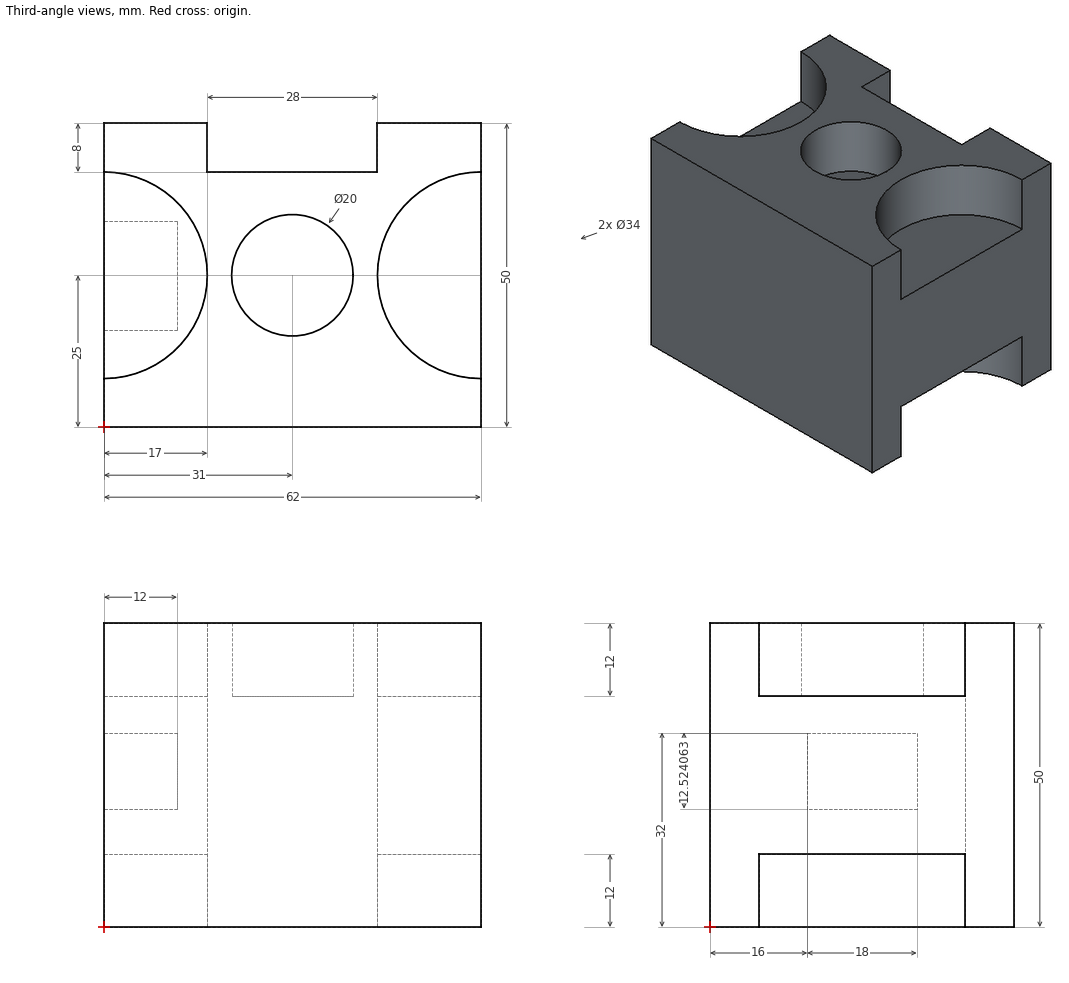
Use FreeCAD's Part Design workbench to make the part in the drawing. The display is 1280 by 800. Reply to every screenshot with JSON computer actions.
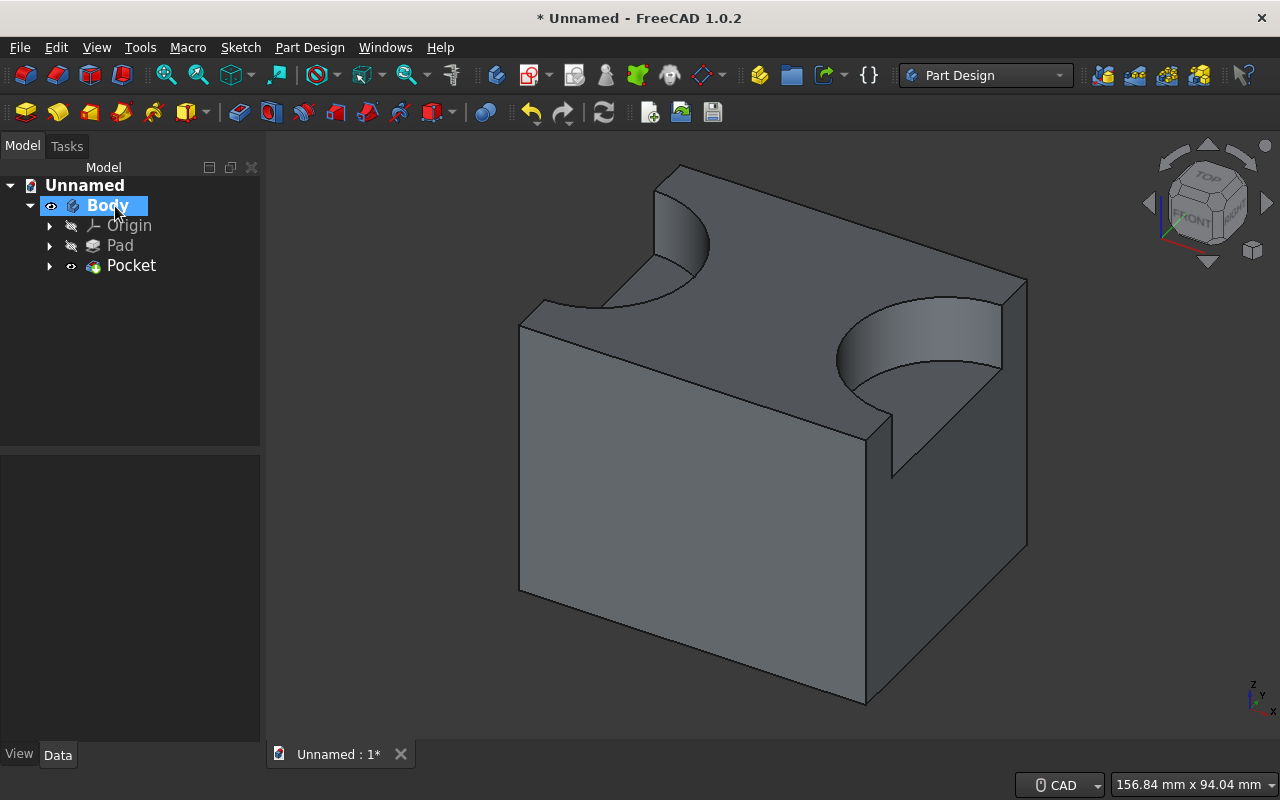
{"action": "left_click", "coordinate": [796, 279]}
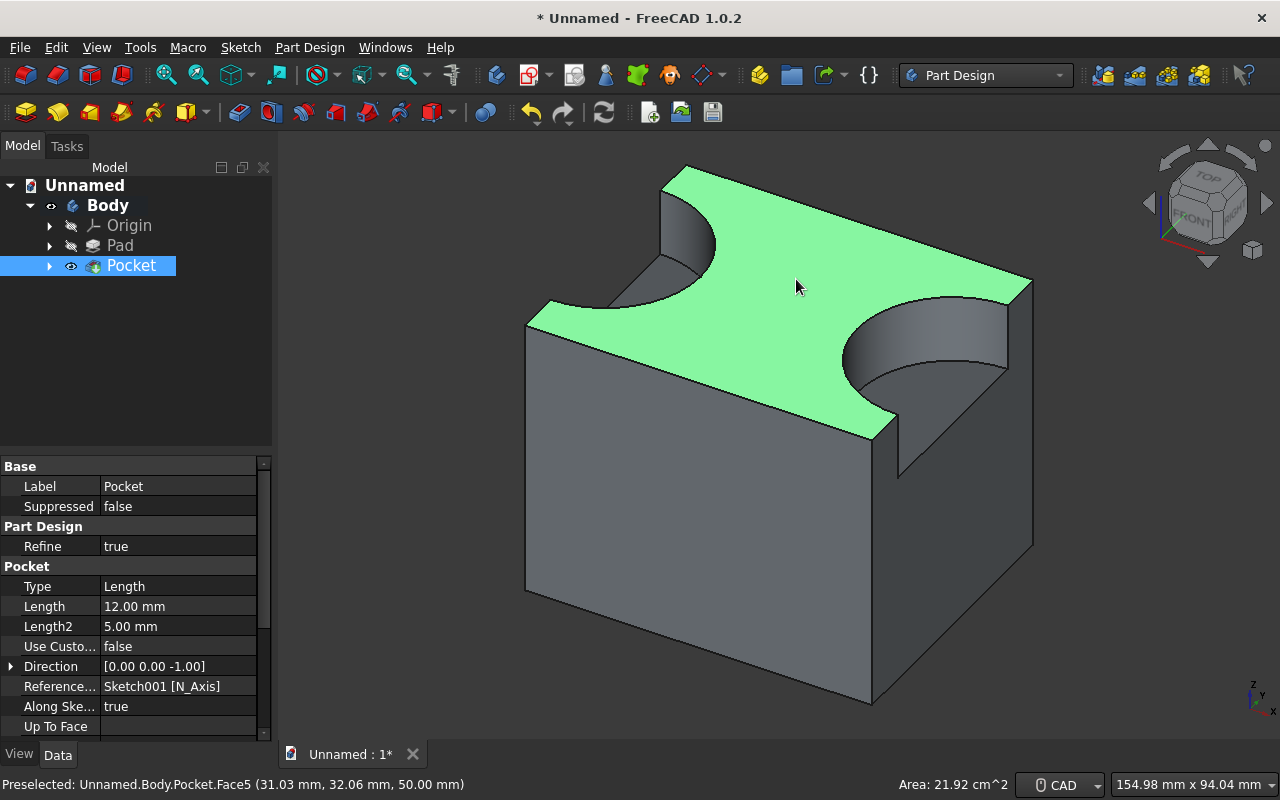
{"action": "left_click", "coordinate": [530, 76]}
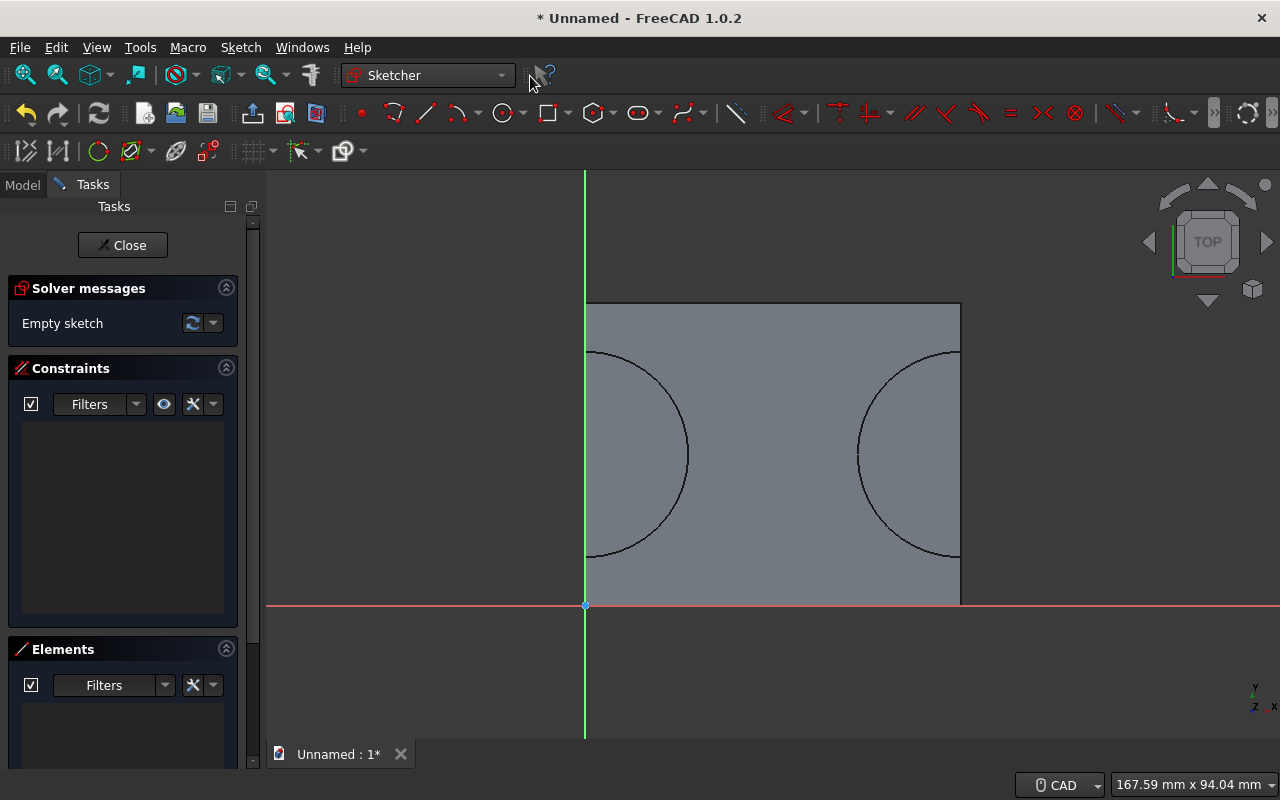
{"action": "left_click", "coordinate": [548, 114]}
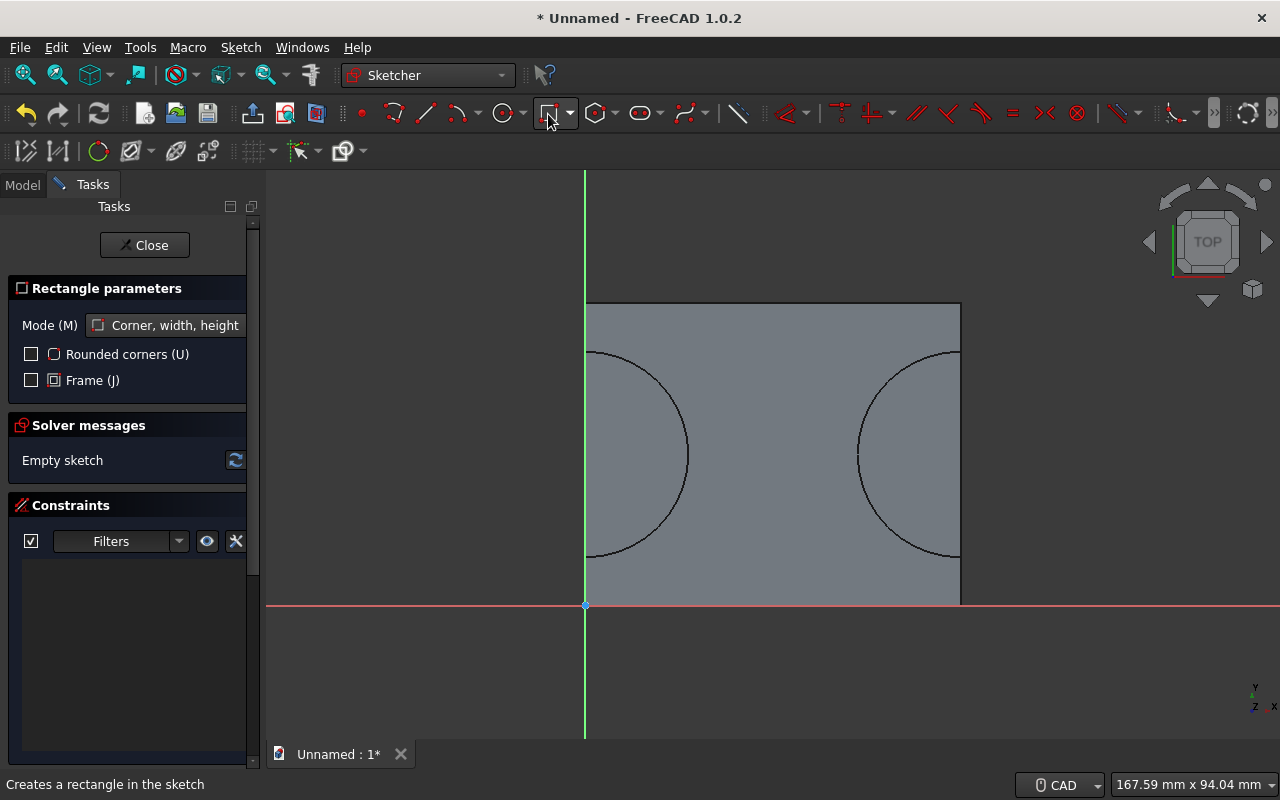
{"action": "left_click", "coordinate": [688, 303]}
{"action": "left_click", "coordinate": [858, 352]}
{"action": "key", "text": "Escape"}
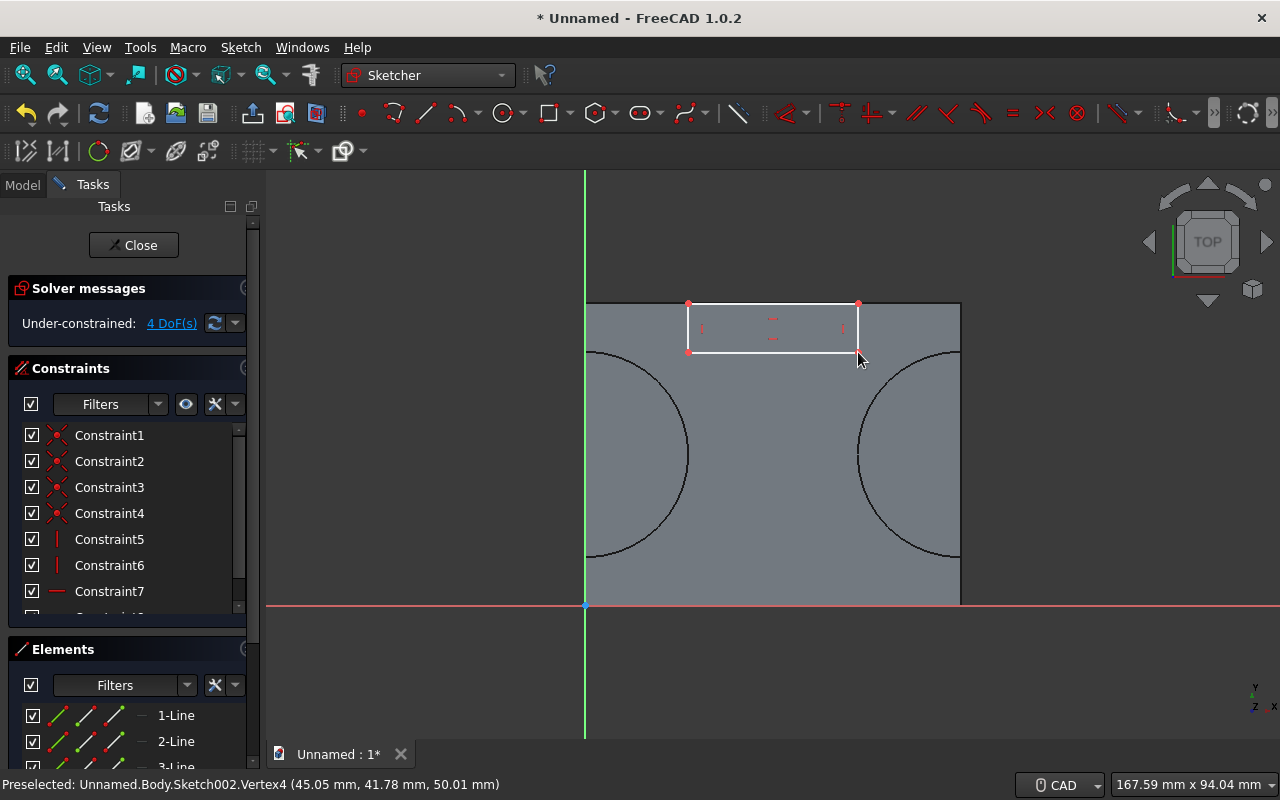
{"action": "left_click", "coordinate": [786, 114]}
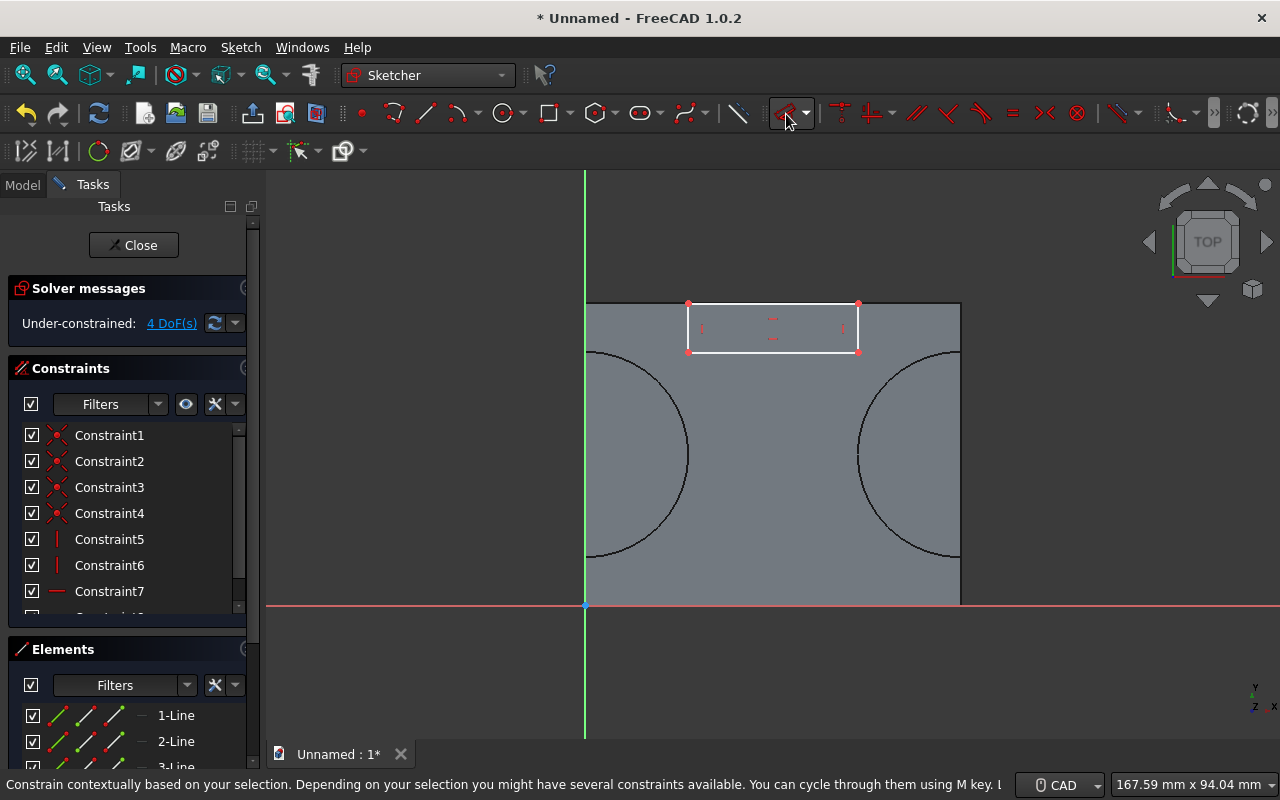
{"action": "left_click", "coordinate": [688, 319]}
{"action": "left_click", "coordinate": [654, 329]}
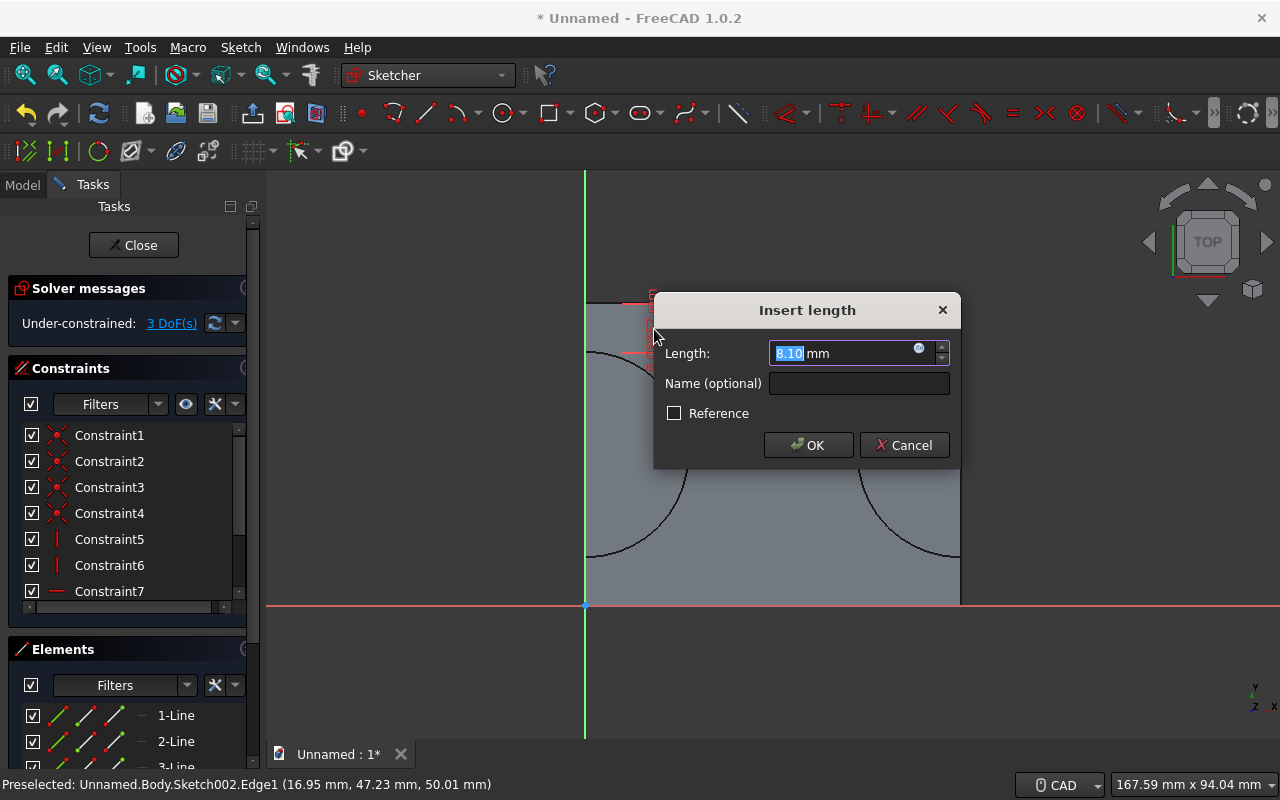
{"action": "type", "text": "8"}
{"action": "key", "text": "Return"}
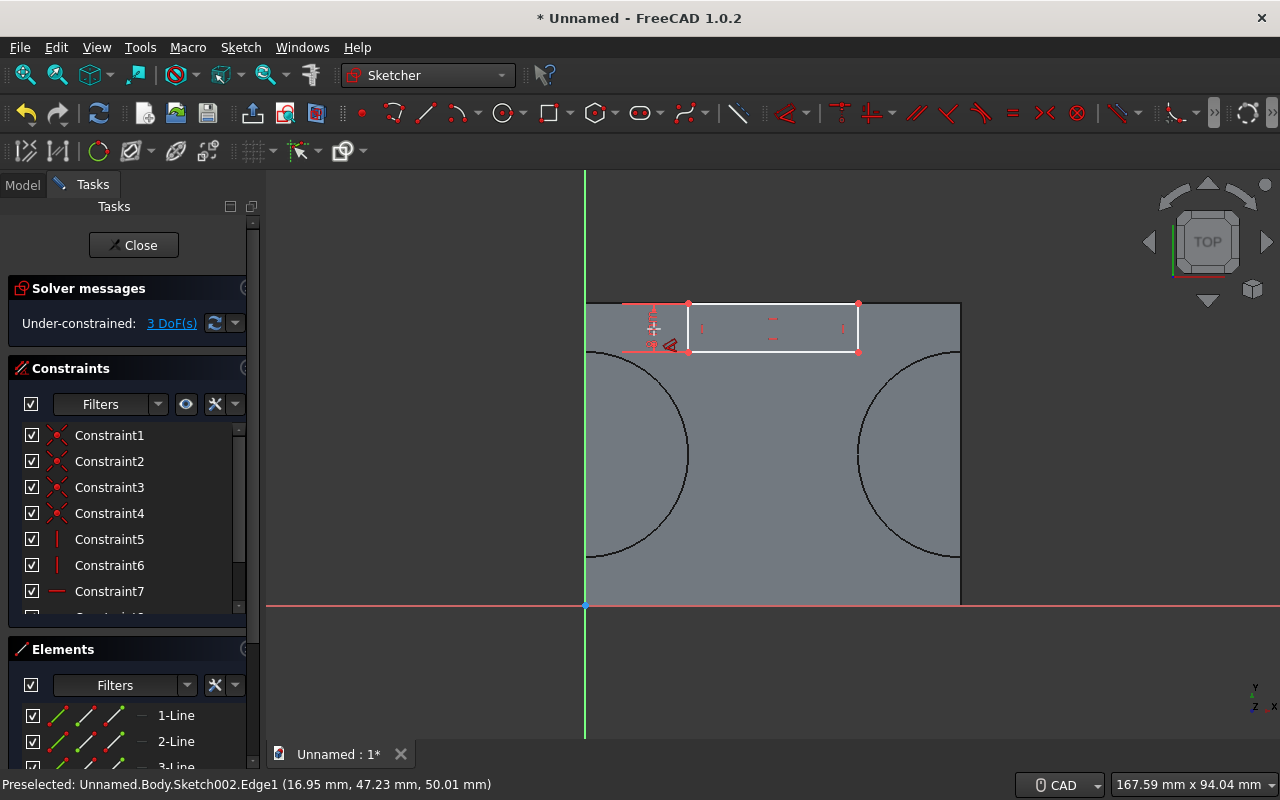
{"action": "left_click", "coordinate": [739, 352]}
{"action": "left_click", "coordinate": [773, 318]}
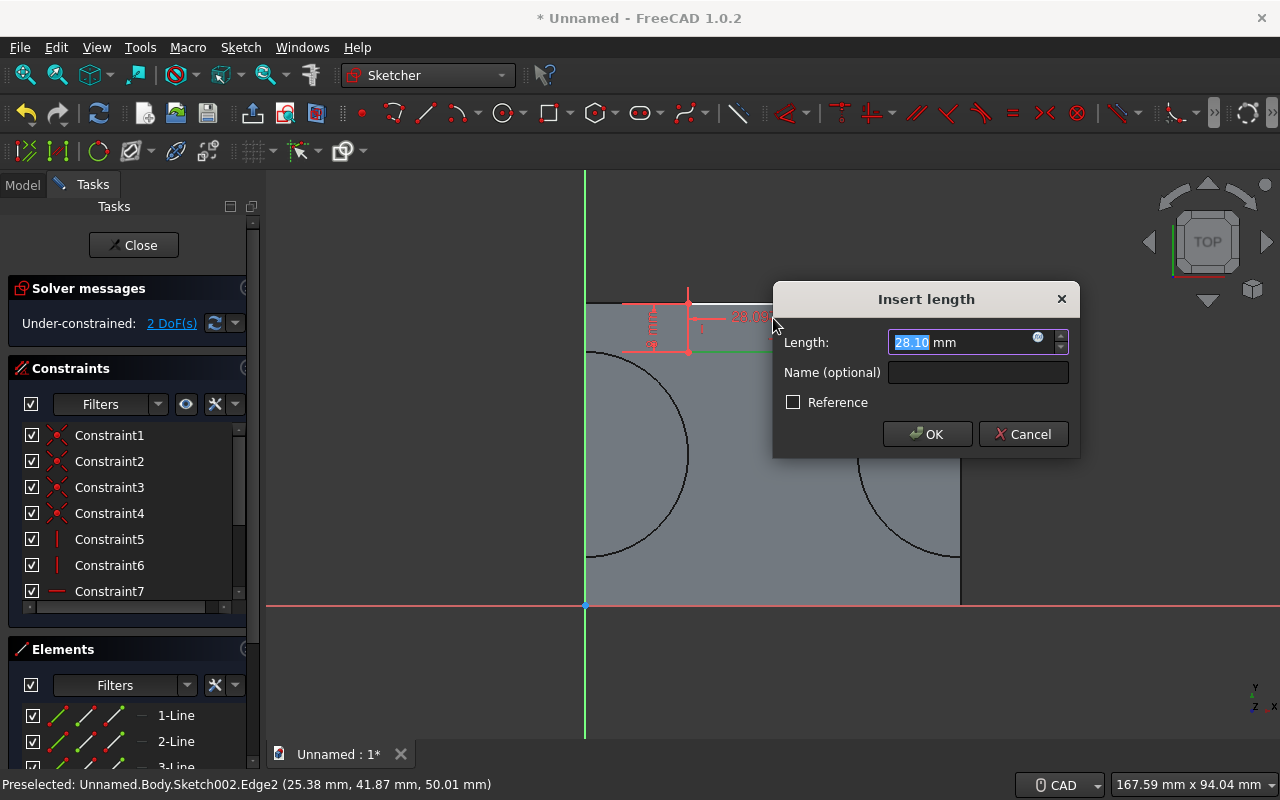
{"action": "type", "text": "28"}
{"action": "key", "text": "Return"}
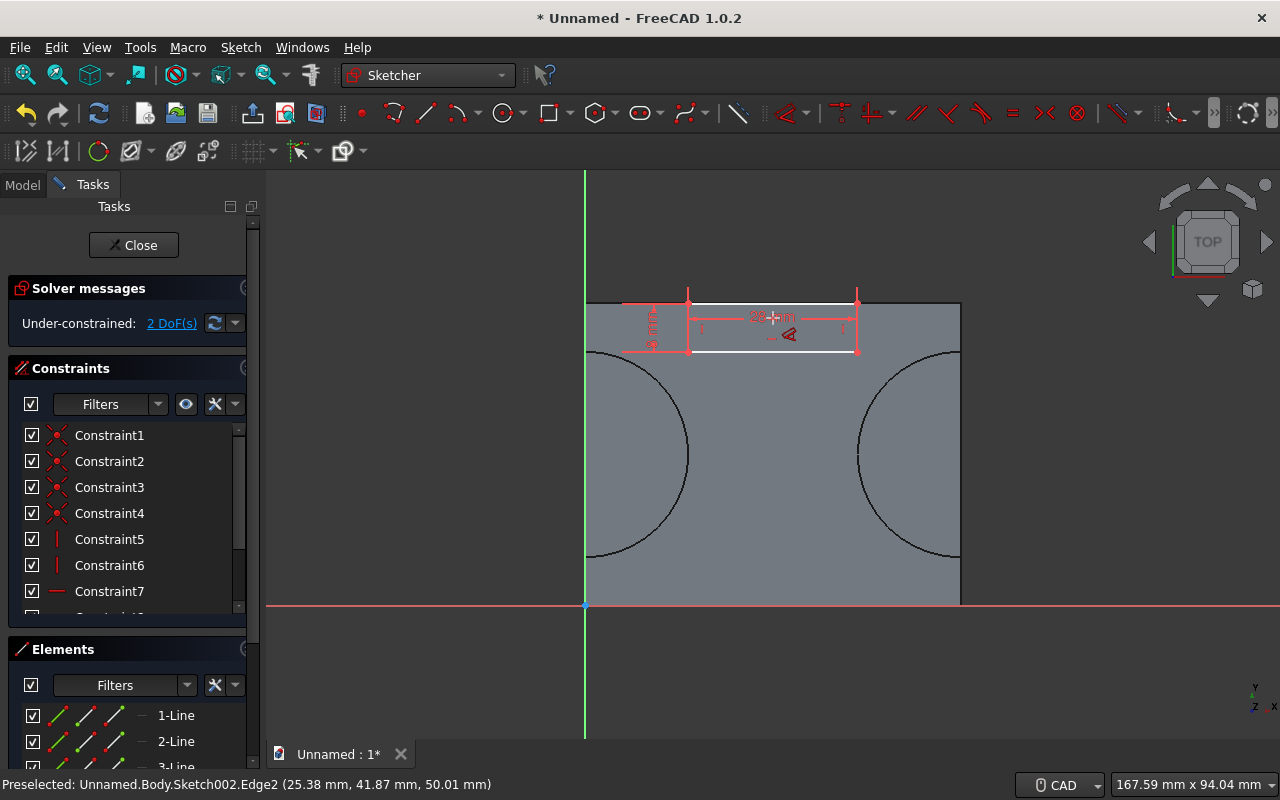
{"action": "left_click", "coordinate": [688, 304]}
{"action": "left_click", "coordinate": [637, 640]}